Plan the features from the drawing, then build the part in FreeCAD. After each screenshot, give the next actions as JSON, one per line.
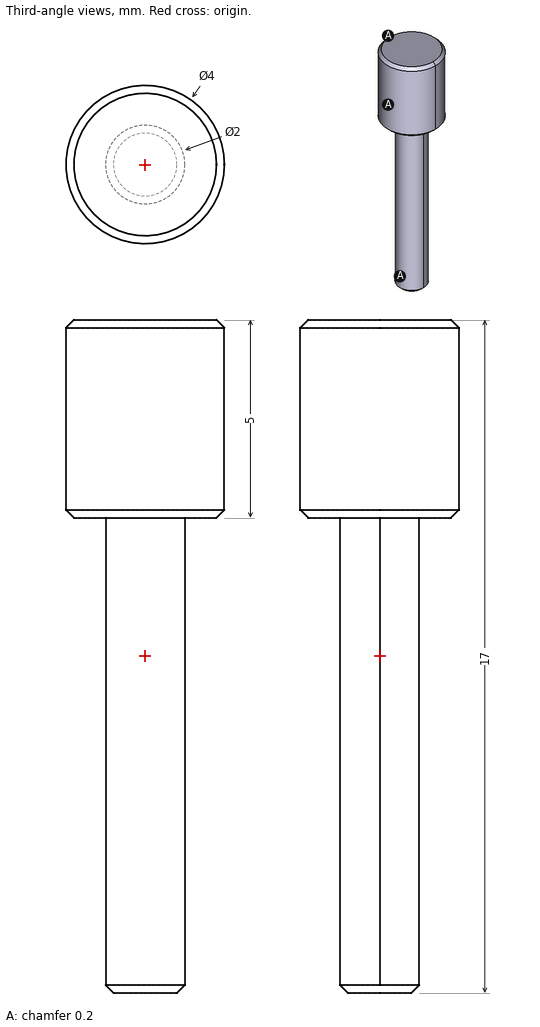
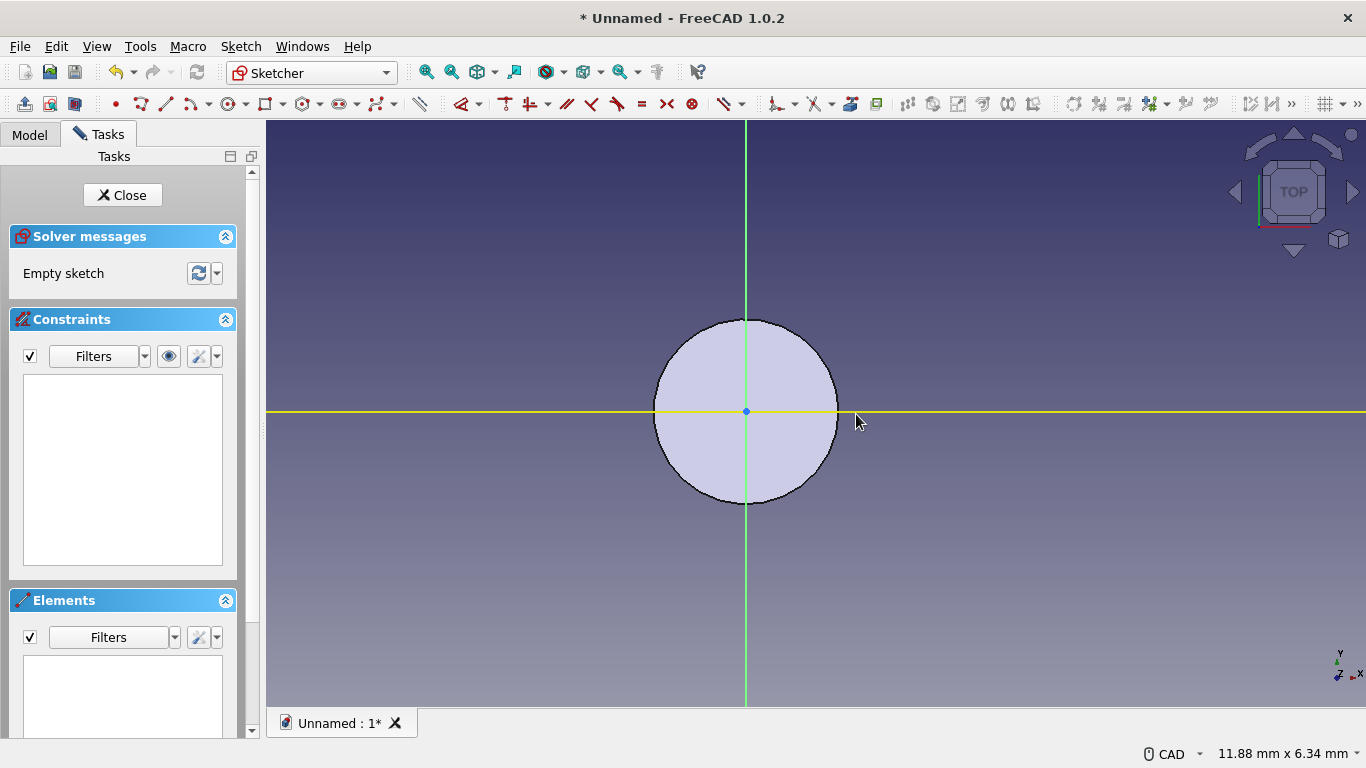
{"action": "left_click", "coordinate": [228, 104]}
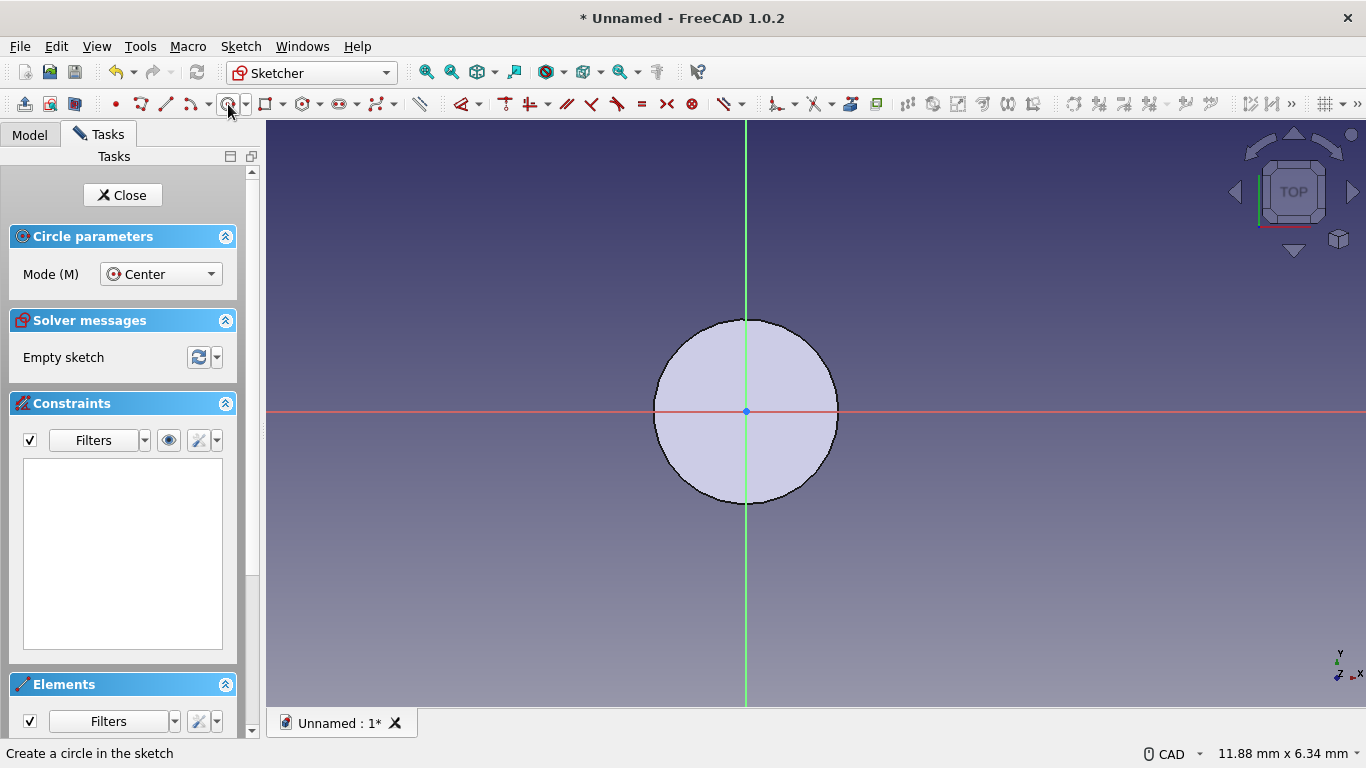
{"action": "left_click", "coordinate": [746, 412]}
{"action": "left_click", "coordinate": [877, 281]}
{"action": "key", "text": "Escape"}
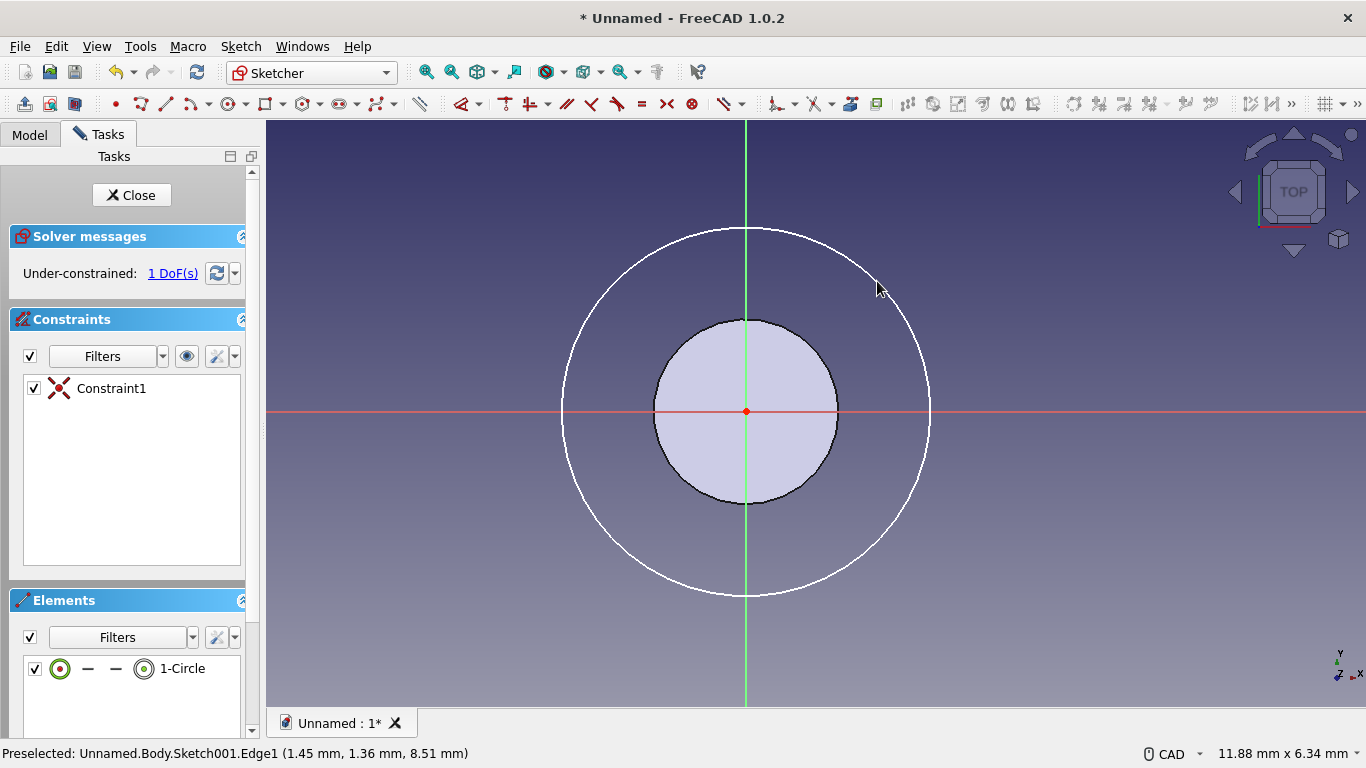
{"action": "left_click", "coordinate": [460, 104]}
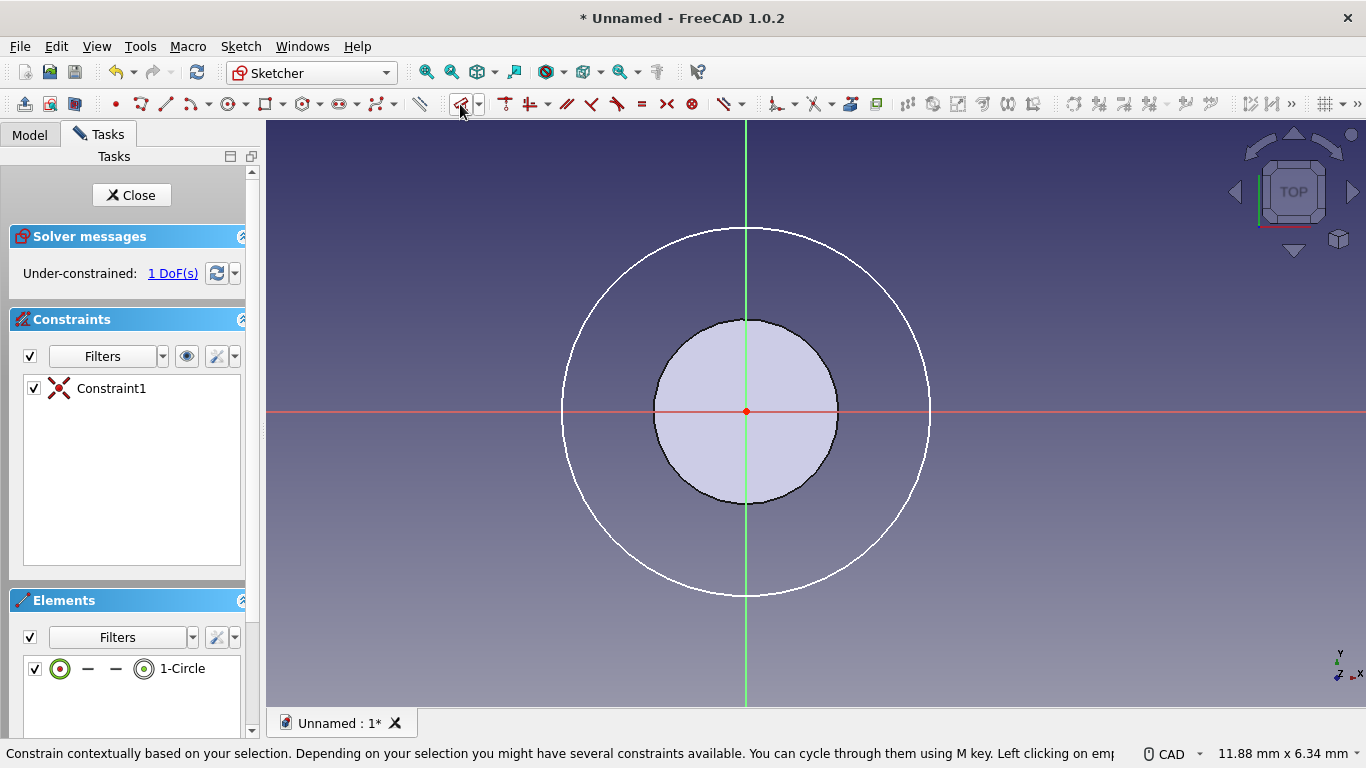
{"action": "left_click", "coordinate": [876, 281]}
{"action": "left_click", "coordinate": [899, 258]}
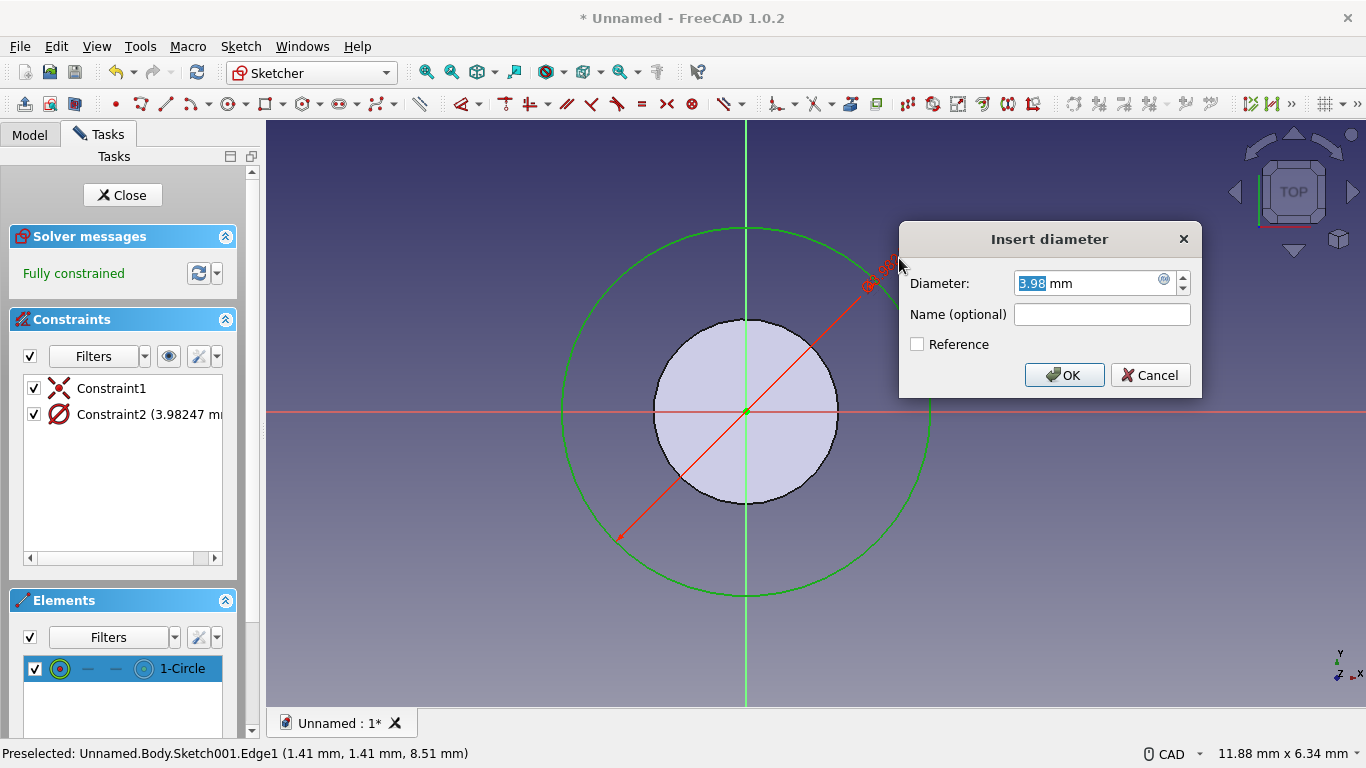
{"action": "type", "text": "4"}
{"action": "key", "text": "Return"}
{"action": "key", "text": "Escape"}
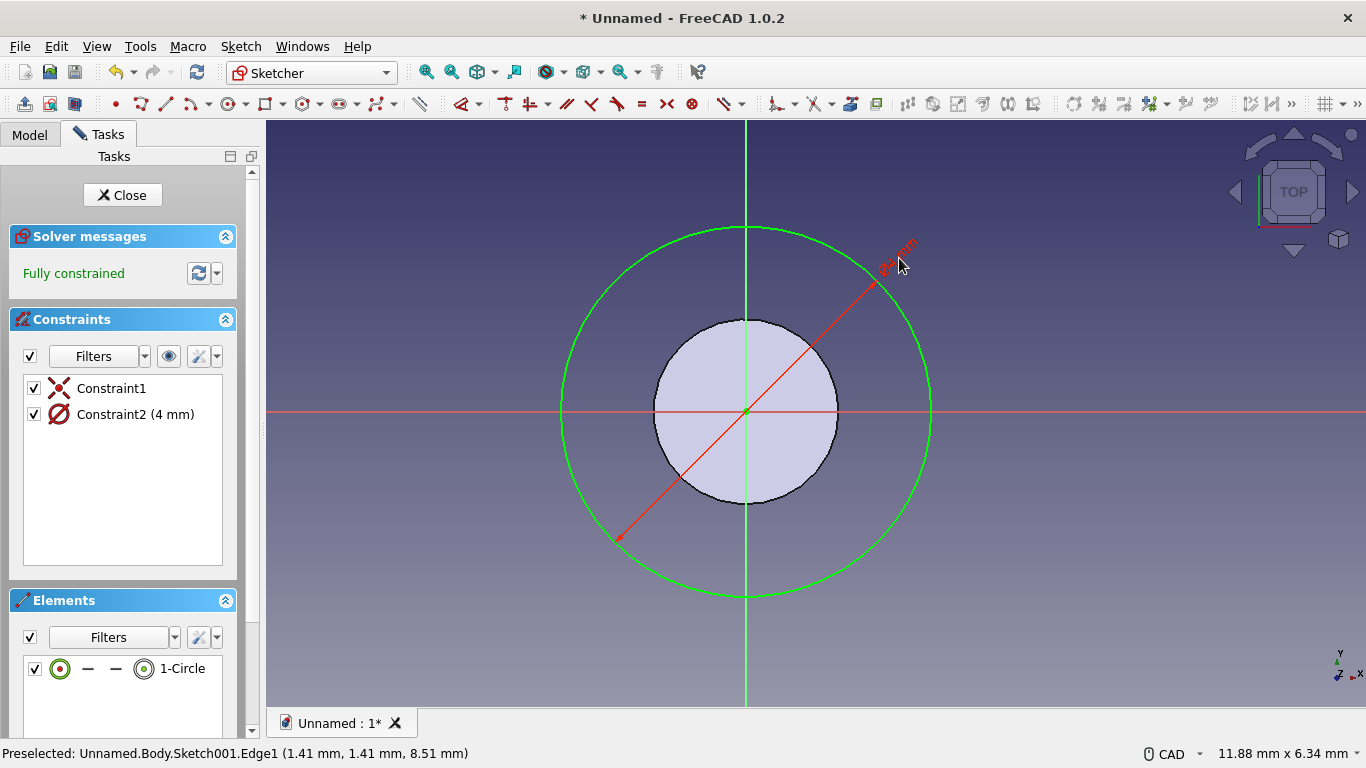
{"action": "left_click", "coordinate": [123, 195]}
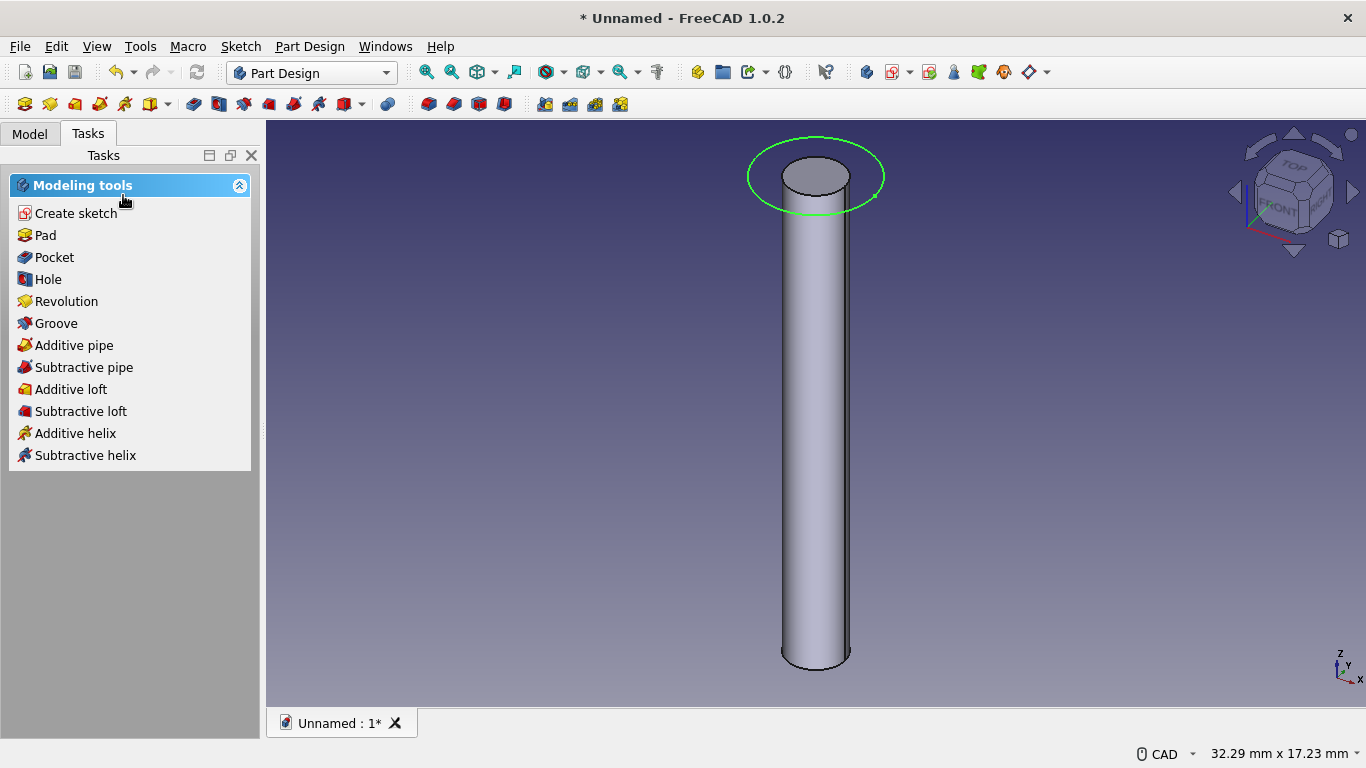
{"action": "left_click", "coordinate": [25, 104]}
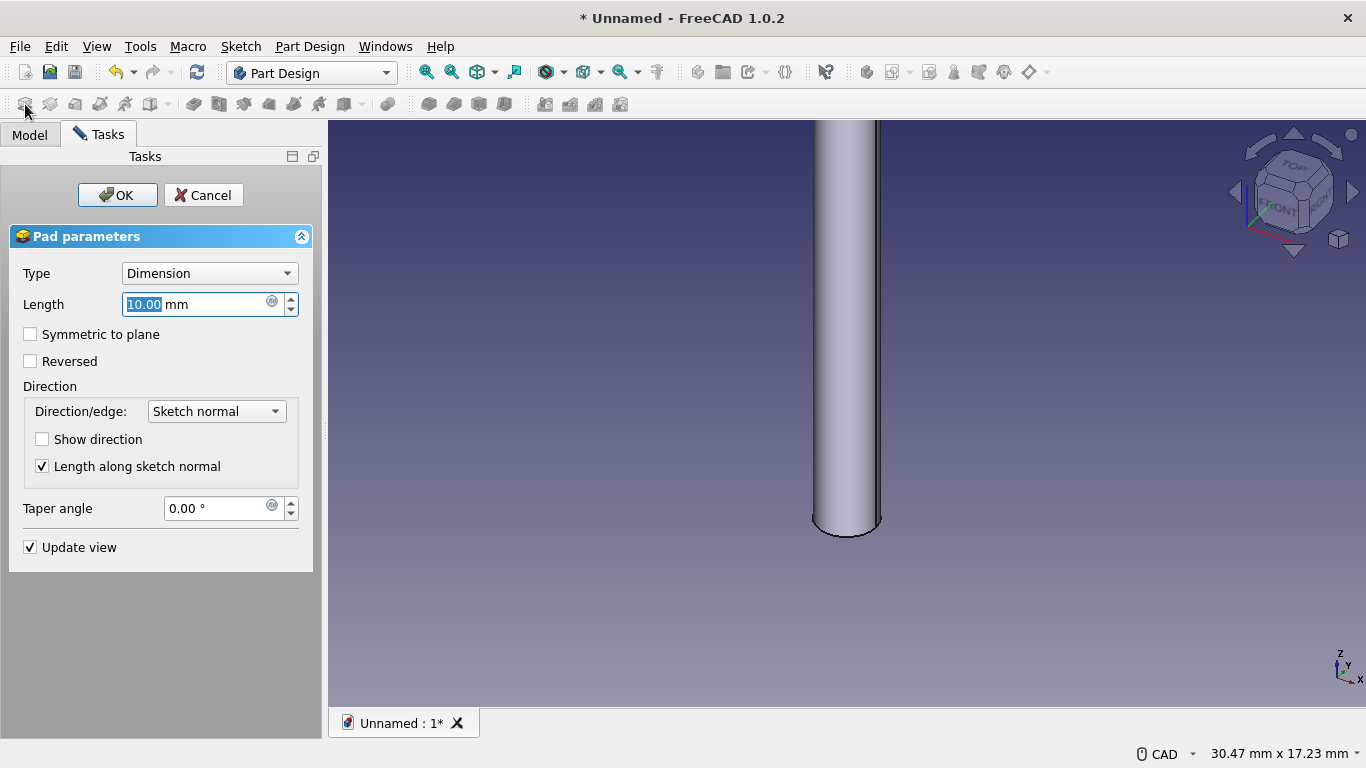
{"action": "type", "text": "5"}
{"action": "key", "text": "Tab"}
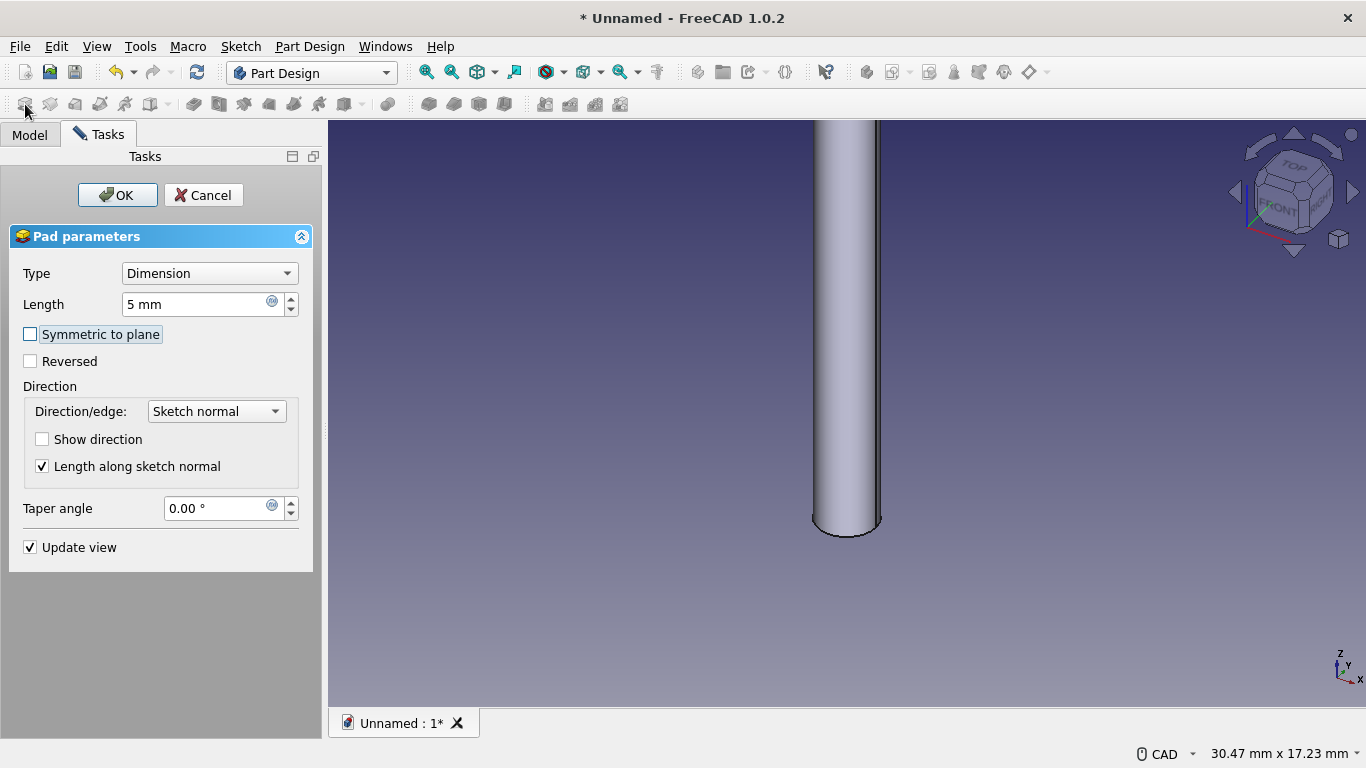
{"action": "left_click", "coordinate": [31, 361]}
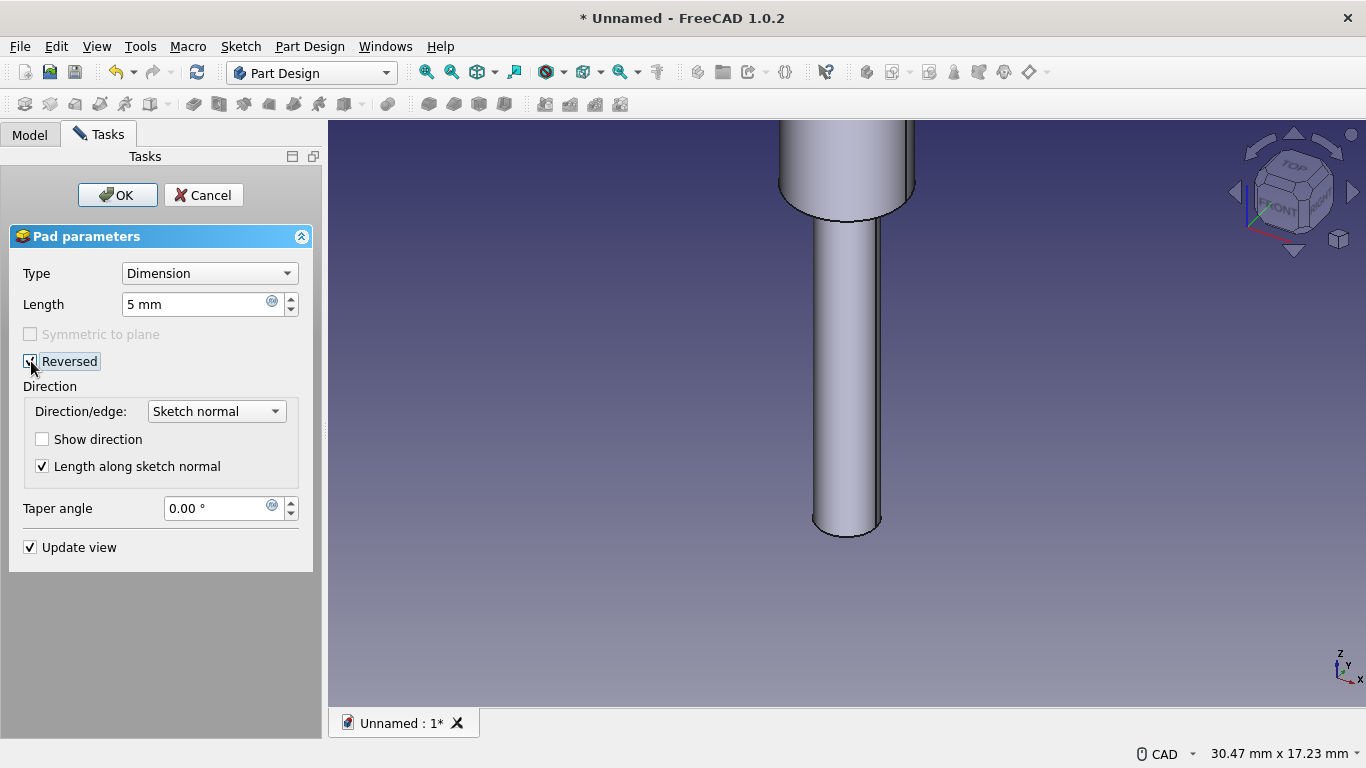
{"action": "left_click", "coordinate": [118, 195]}